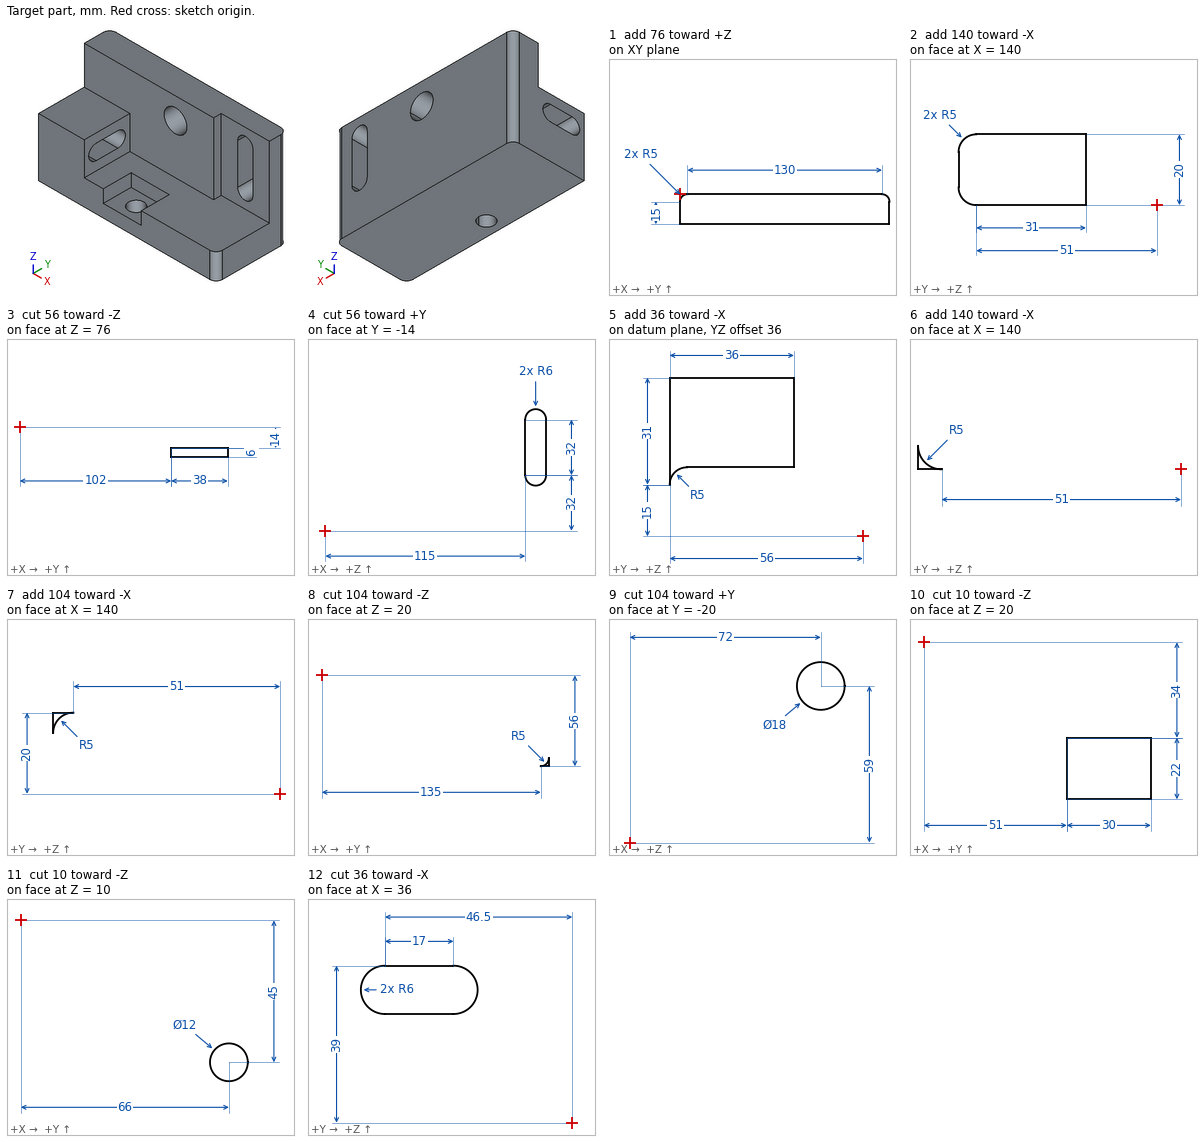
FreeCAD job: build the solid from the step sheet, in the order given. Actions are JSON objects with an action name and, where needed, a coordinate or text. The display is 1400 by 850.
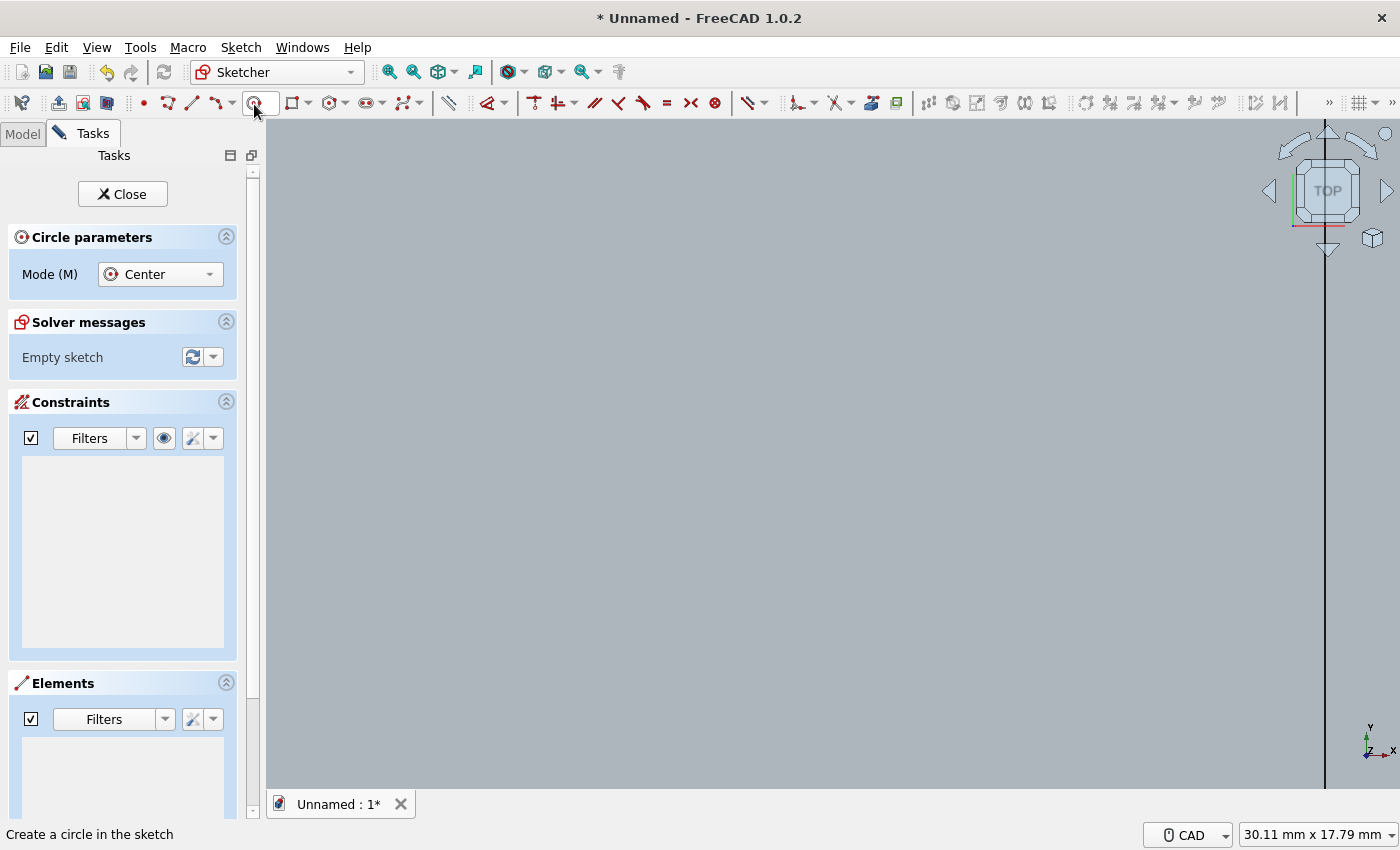
{"action": "left_click", "coordinate": [760, 448]}
{"action": "left_click", "coordinate": [920, 288]}
{"action": "key", "text": "Escape"}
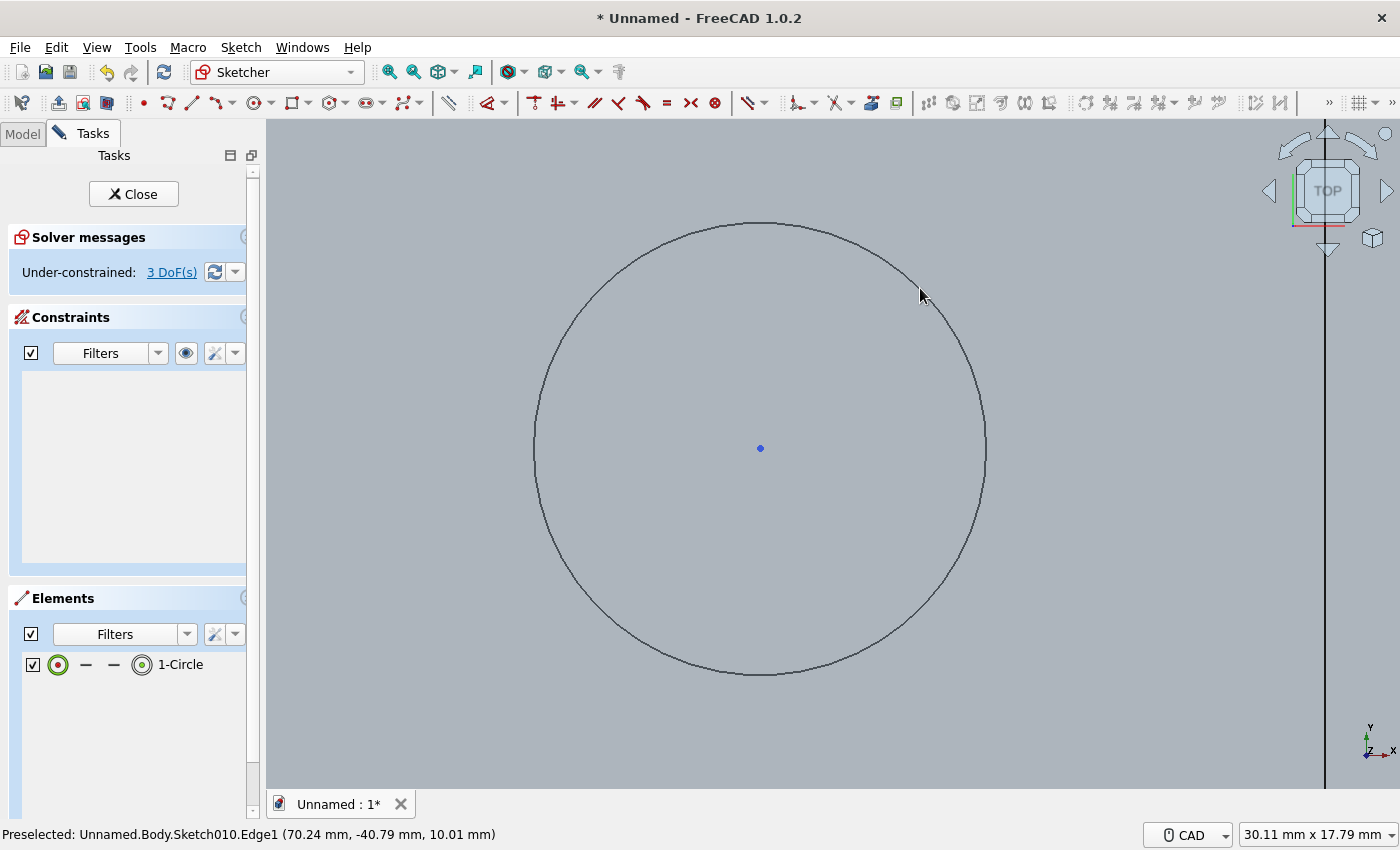
{"action": "left_click", "coordinate": [488, 104]}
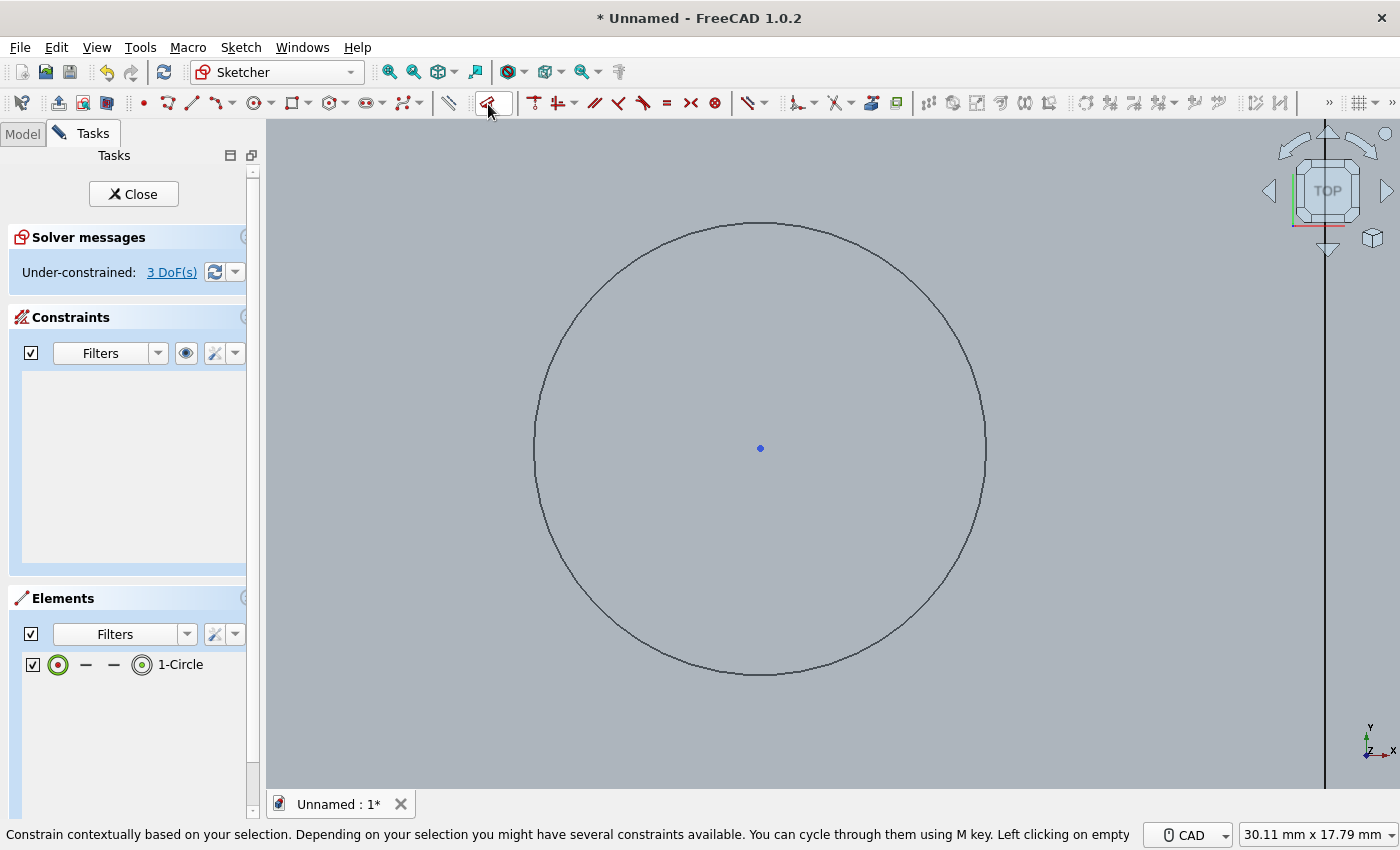
{"action": "left_click", "coordinate": [920, 289]}
{"action": "left_click", "coordinate": [943, 266]}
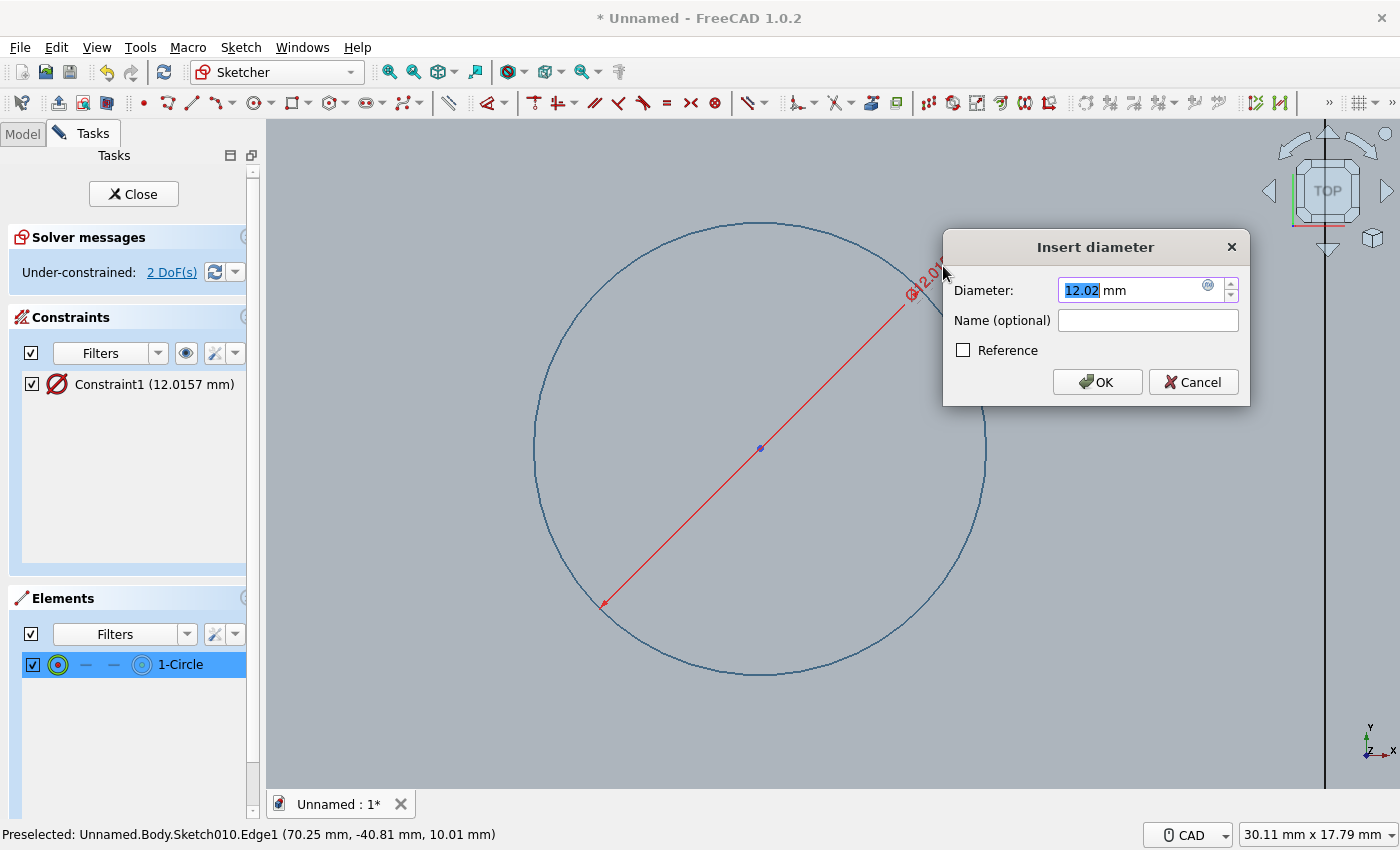
{"action": "type", "text": "12"}
{"action": "key", "text": "Return"}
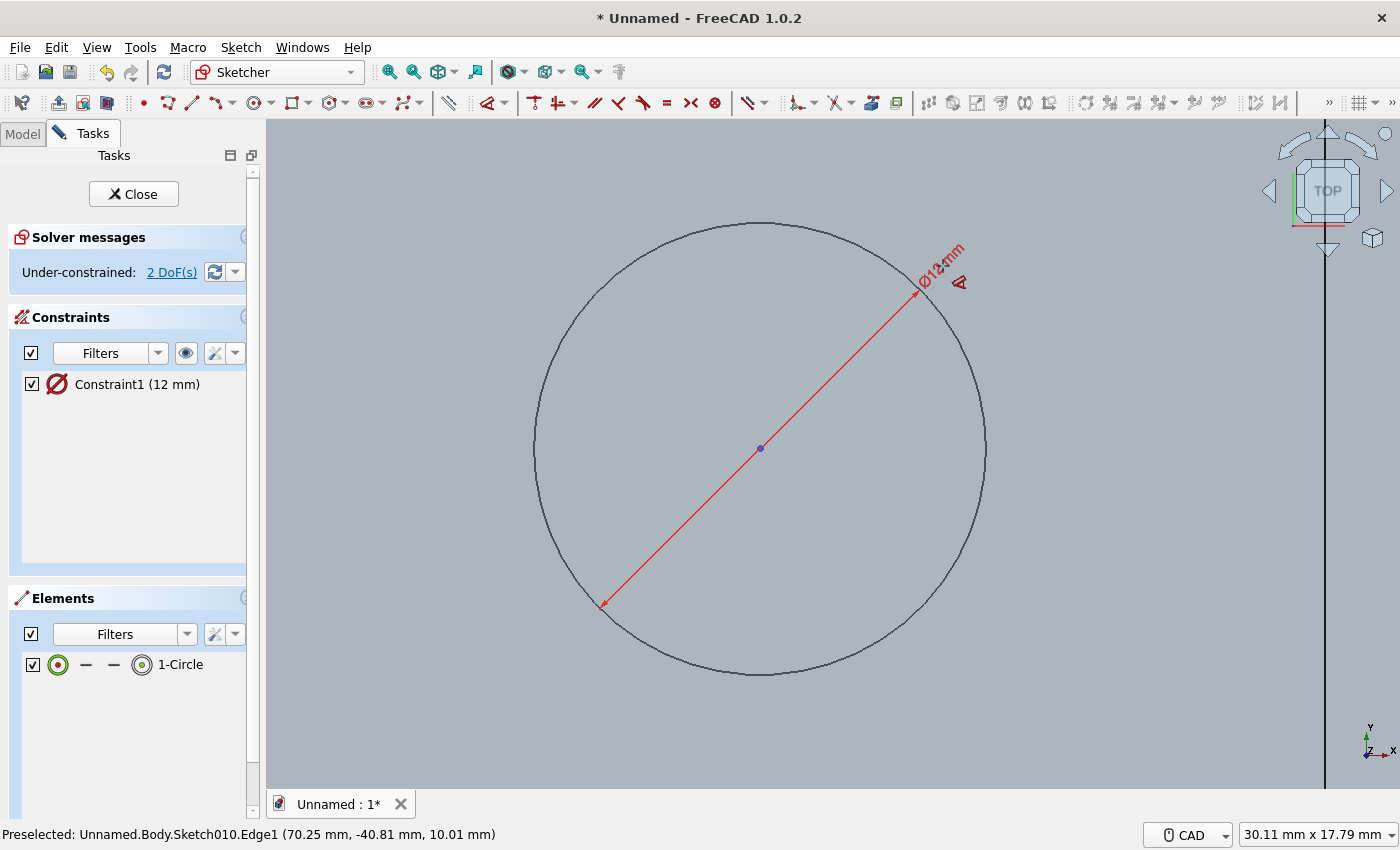
{"action": "left_click", "coordinate": [760, 449]}
{"action": "left_click", "coordinate": [420, 483]}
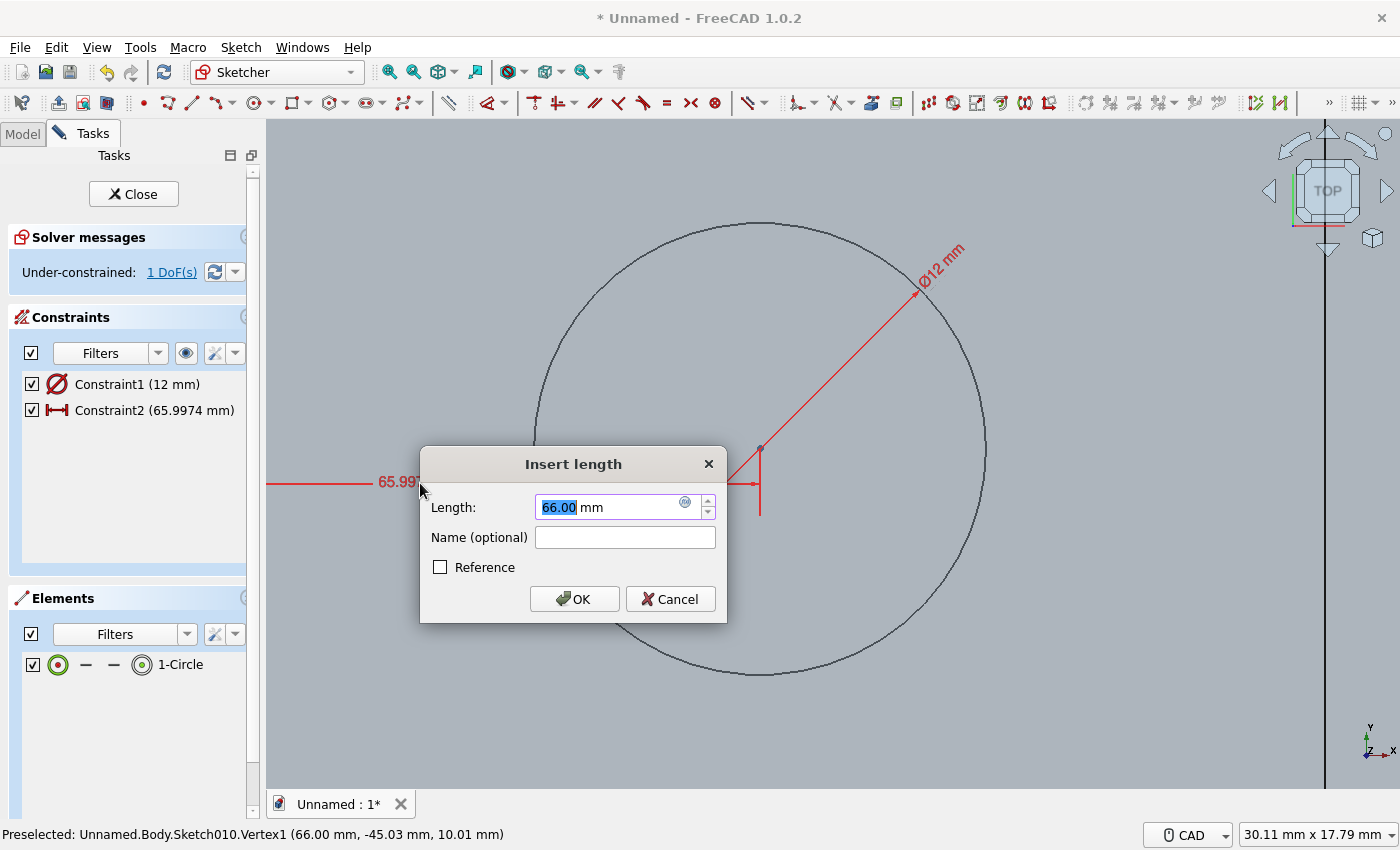
{"action": "type", "text": "66"}
{"action": "key", "text": "Return"}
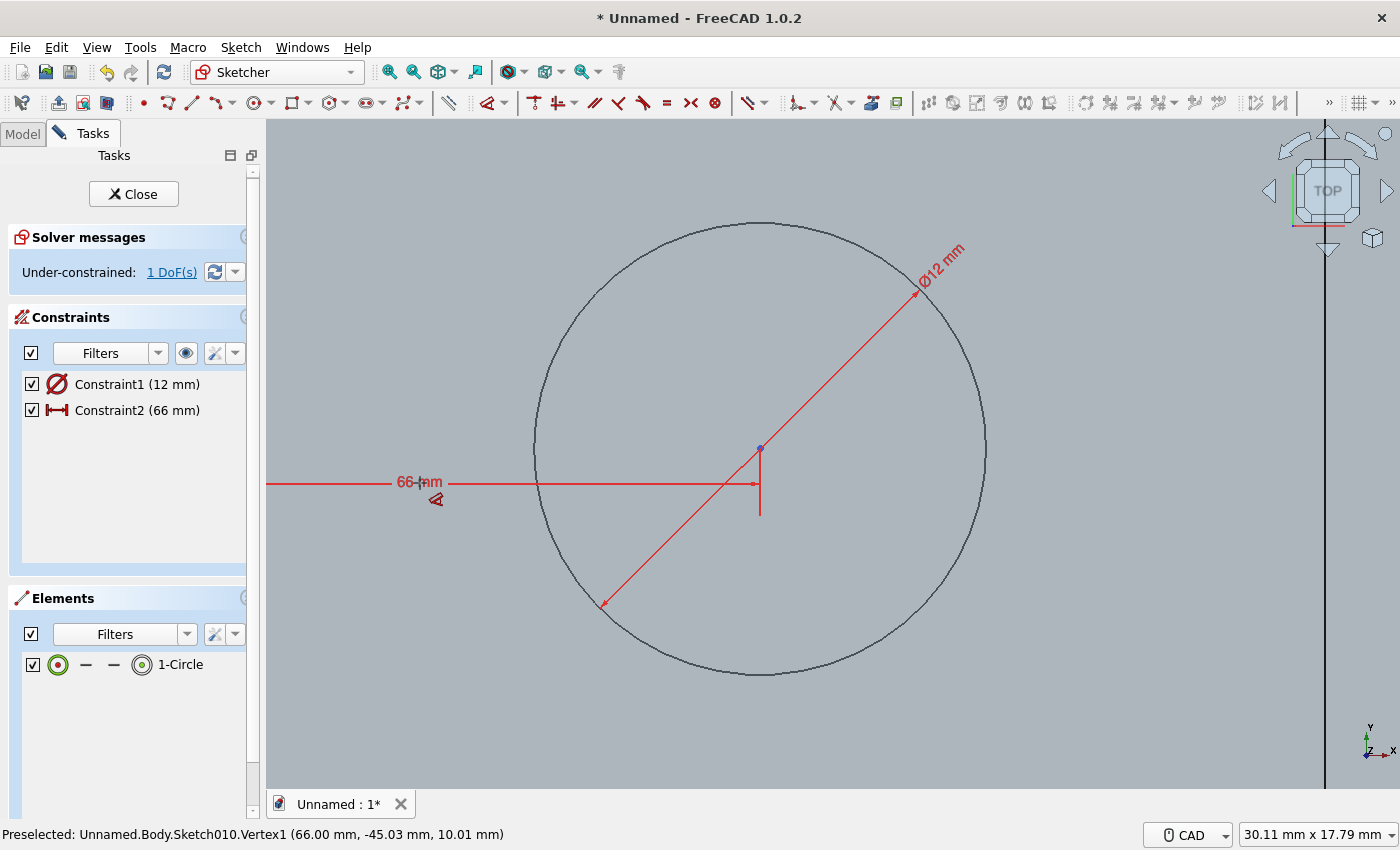
{"action": "left_click", "coordinate": [760, 449]}
{"action": "left_click", "coordinate": [794, 298]}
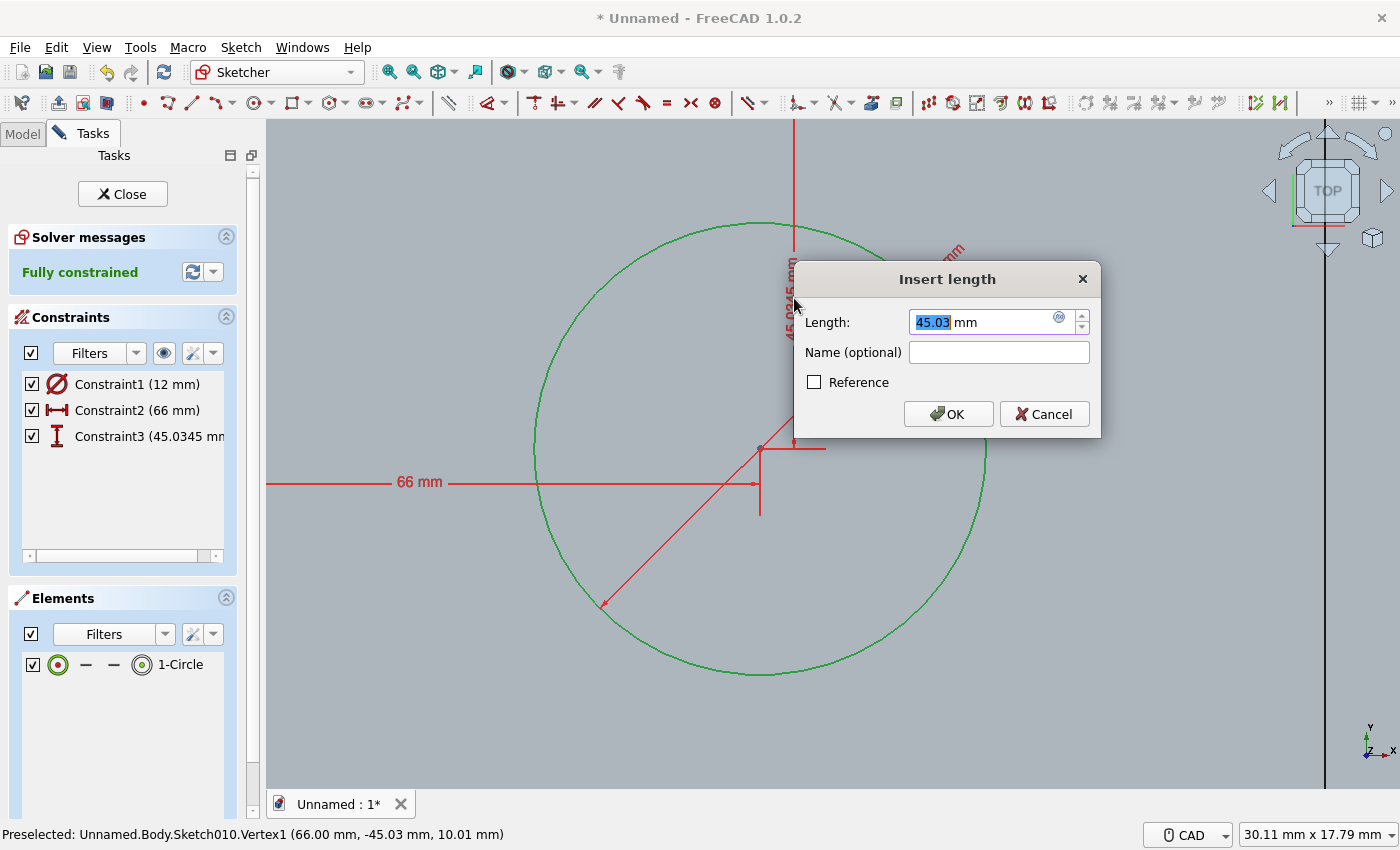
{"action": "type", "text": "45"}
{"action": "key", "text": "Return"}
{"action": "key", "text": "Escape"}